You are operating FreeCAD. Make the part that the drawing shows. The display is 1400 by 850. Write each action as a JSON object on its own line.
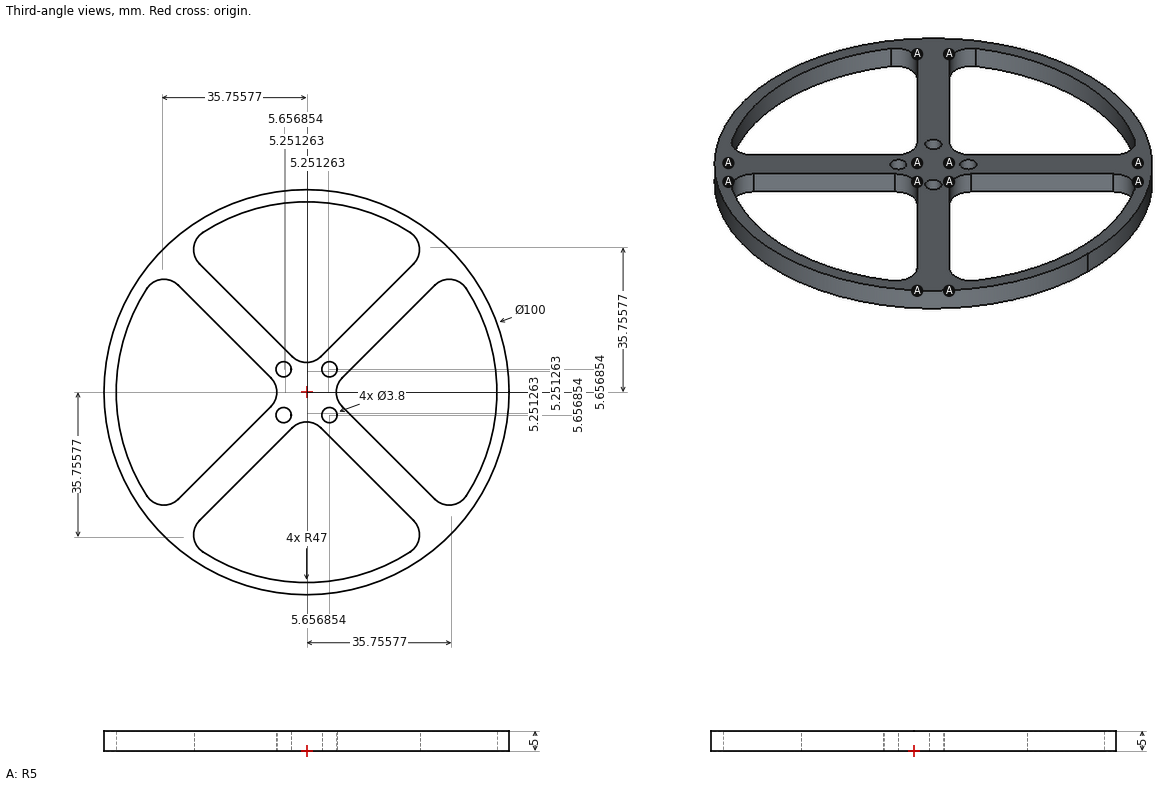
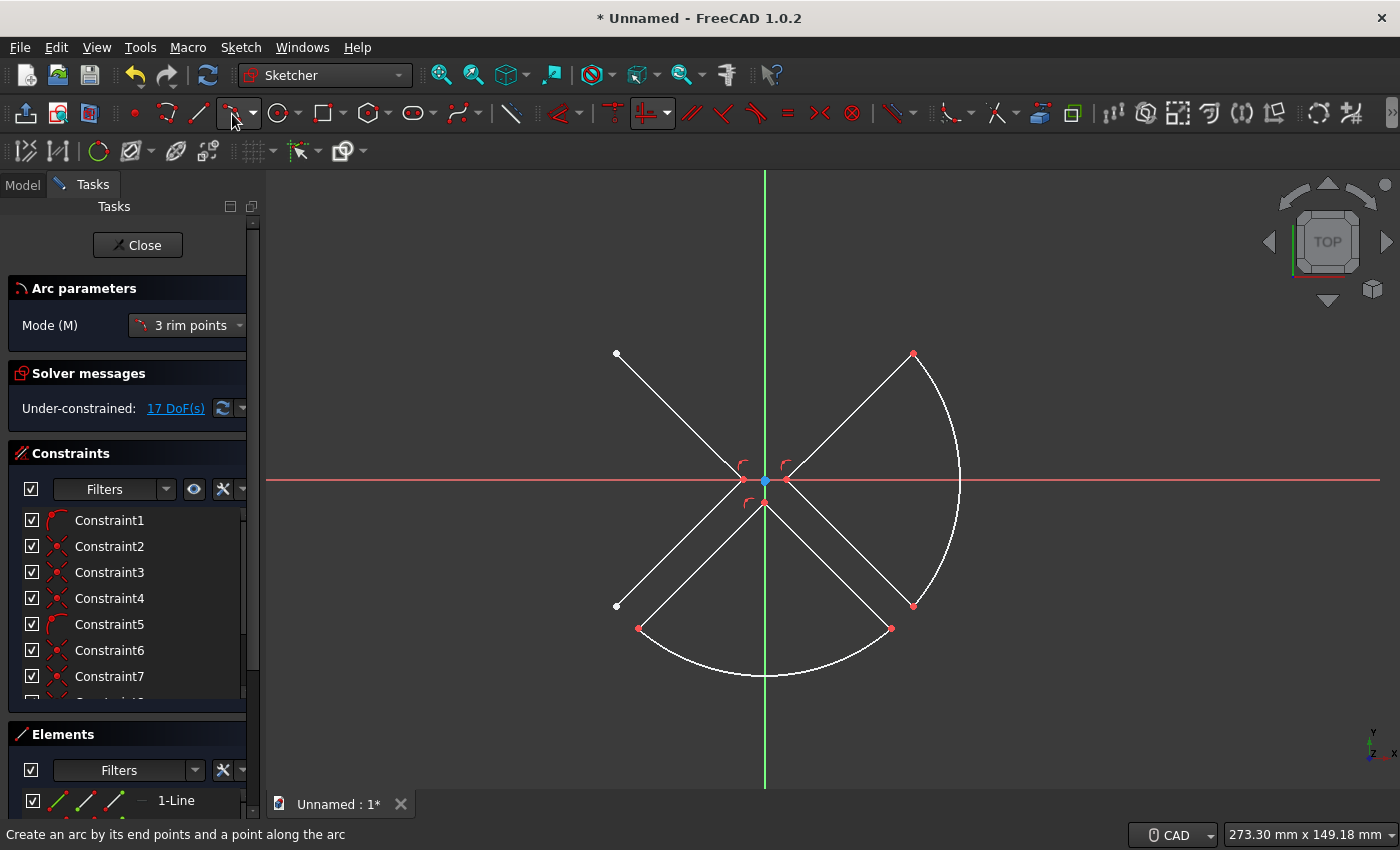
{"action": "left_click", "coordinate": [616, 607]}
{"action": "left_click", "coordinate": [616, 354]}
{"action": "left_click", "coordinate": [571, 452]}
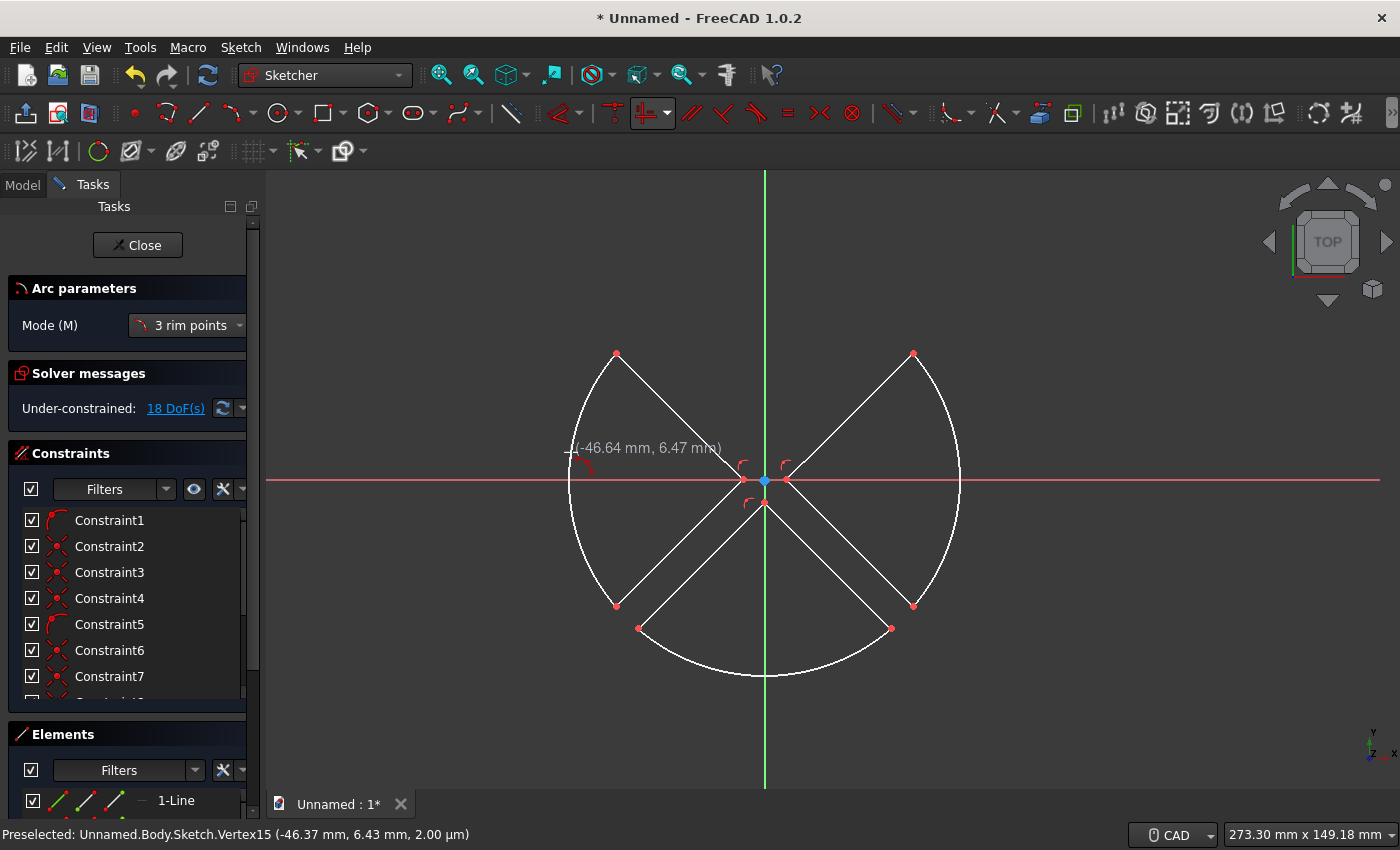
{"action": "left_click", "coordinate": [168, 114]}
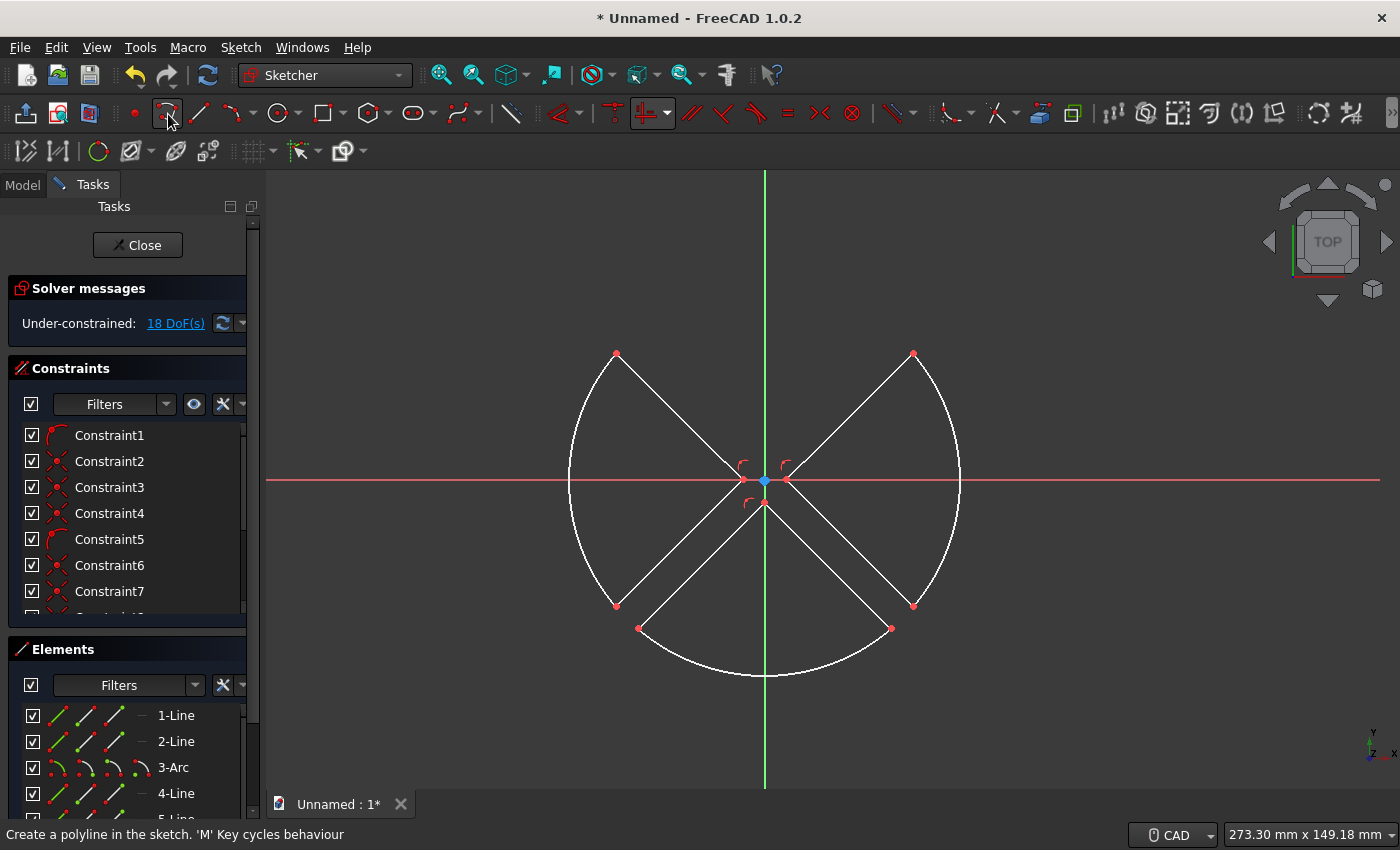
{"action": "left_click", "coordinate": [891, 331]}
{"action": "left_click", "coordinate": [765, 458]}
{"action": "left_click", "coordinate": [638, 331]}
{"action": "right_click", "coordinate": [638, 331]}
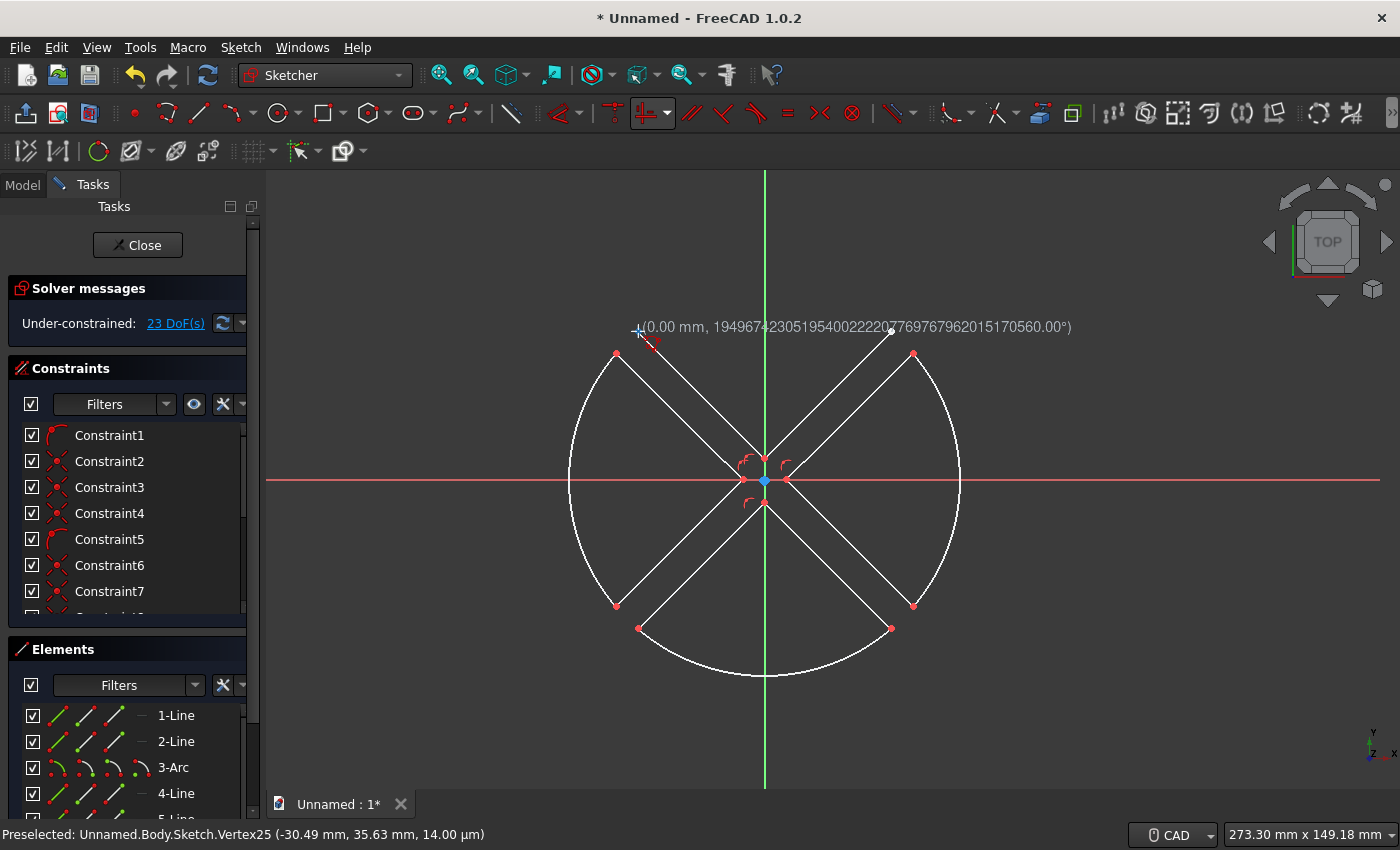
{"action": "left_click", "coordinate": [232, 114]}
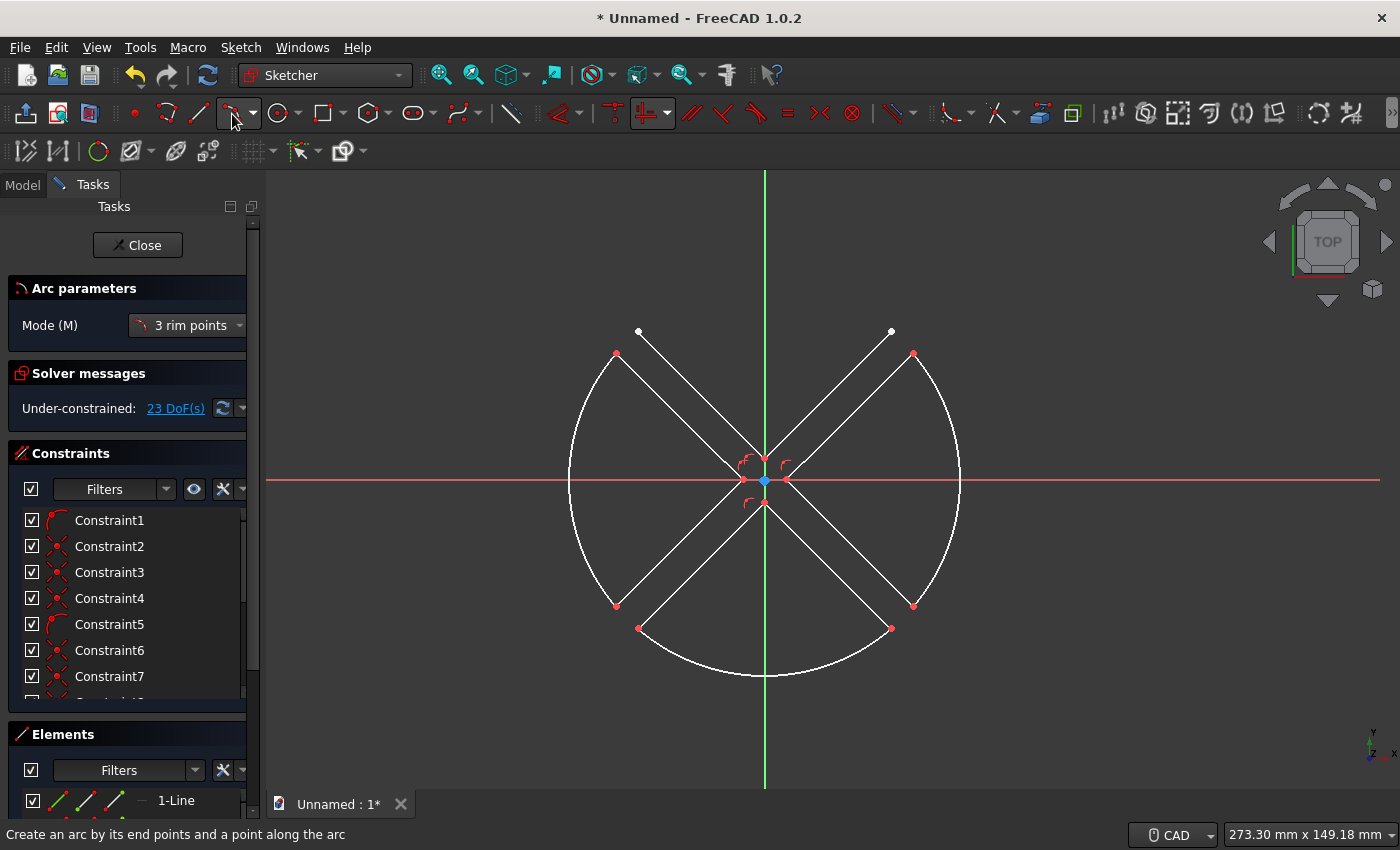
{"action": "left_click", "coordinate": [638, 332]}
{"action": "left_click", "coordinate": [891, 332]}
{"action": "left_click", "coordinate": [792, 287]}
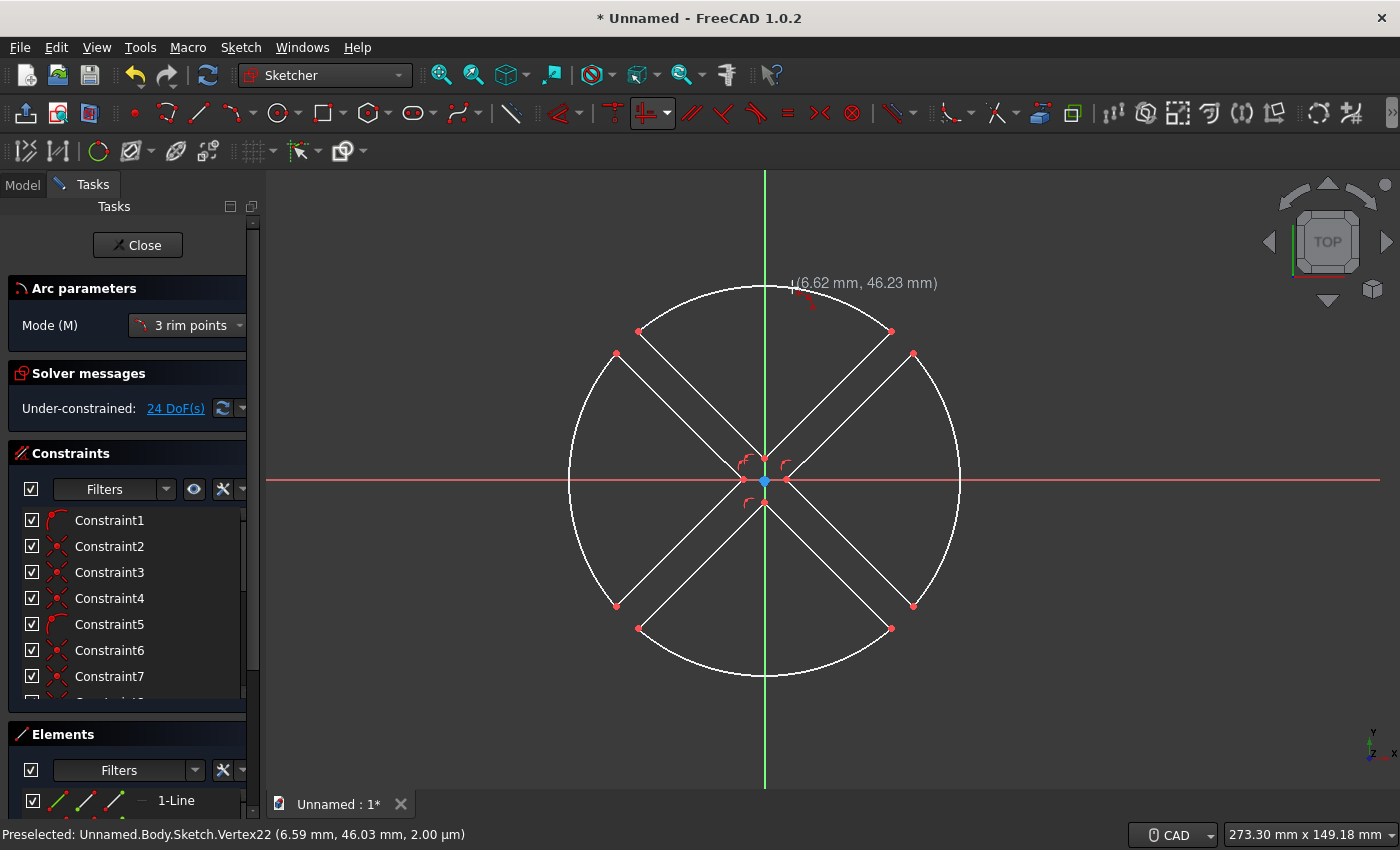
{"action": "left_click", "coordinate": [278, 114]}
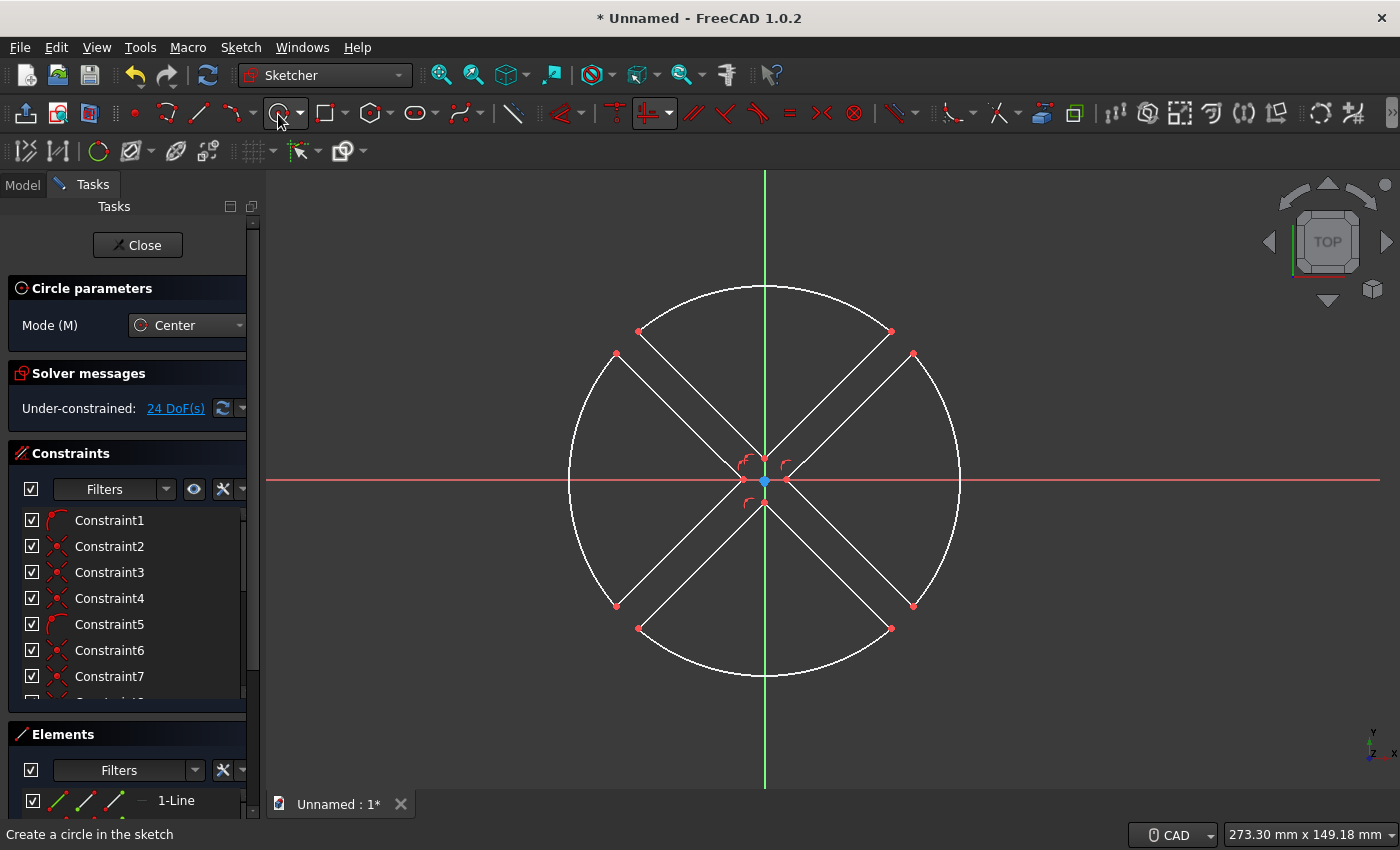
{"action": "left_click", "coordinate": [765, 480]}
{"action": "mouse_move", "coordinate": [911, 333]}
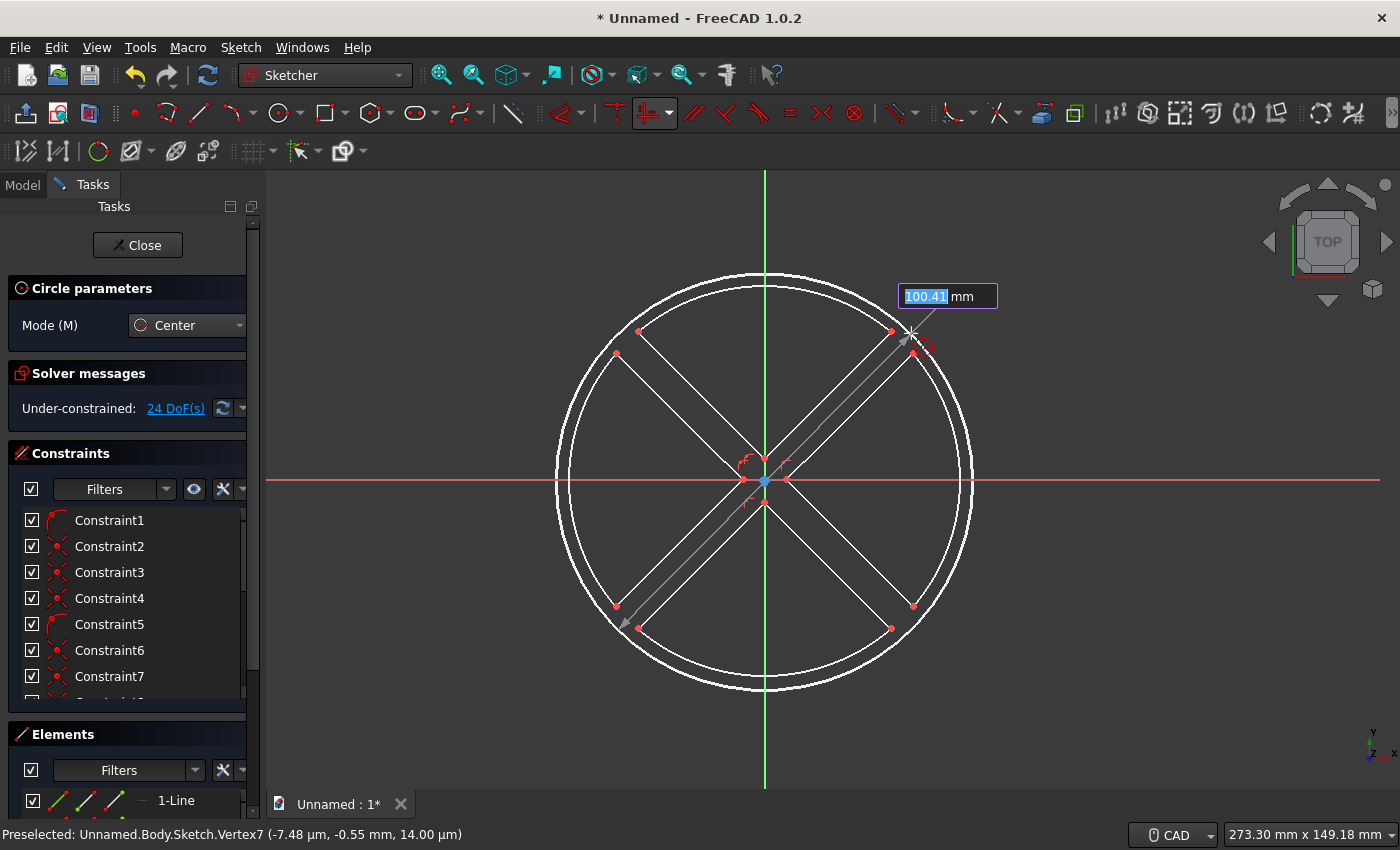
{"action": "type", "text": "100"}
{"action": "key", "text": "Return"}
{"action": "key", "text": "Escape"}